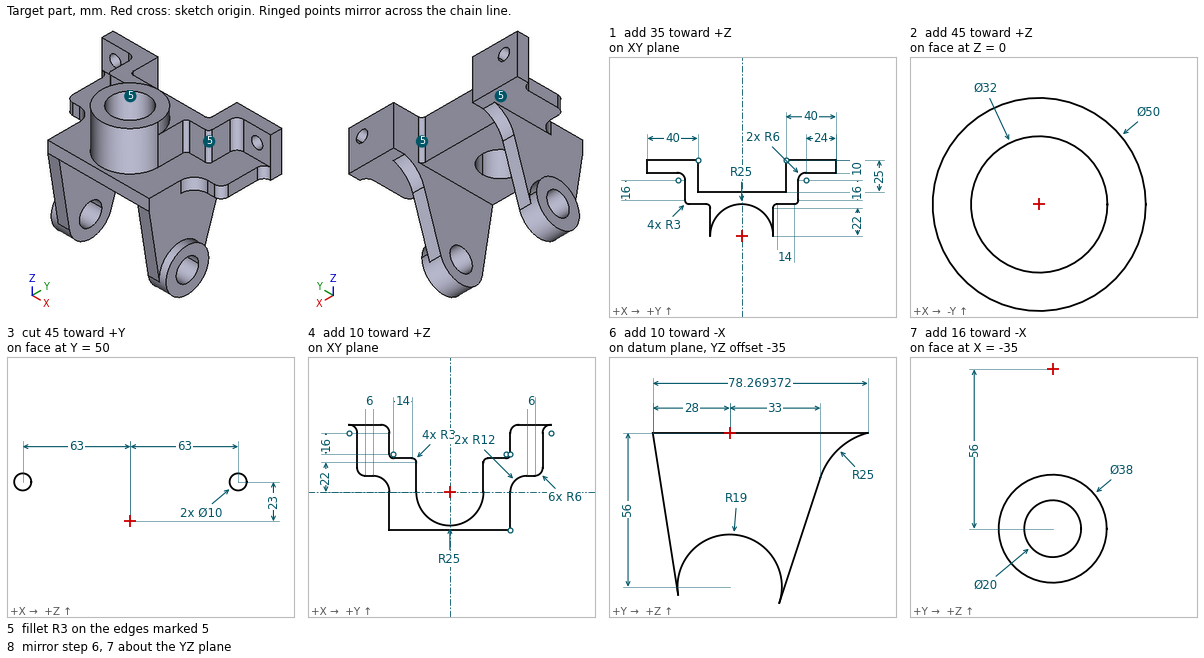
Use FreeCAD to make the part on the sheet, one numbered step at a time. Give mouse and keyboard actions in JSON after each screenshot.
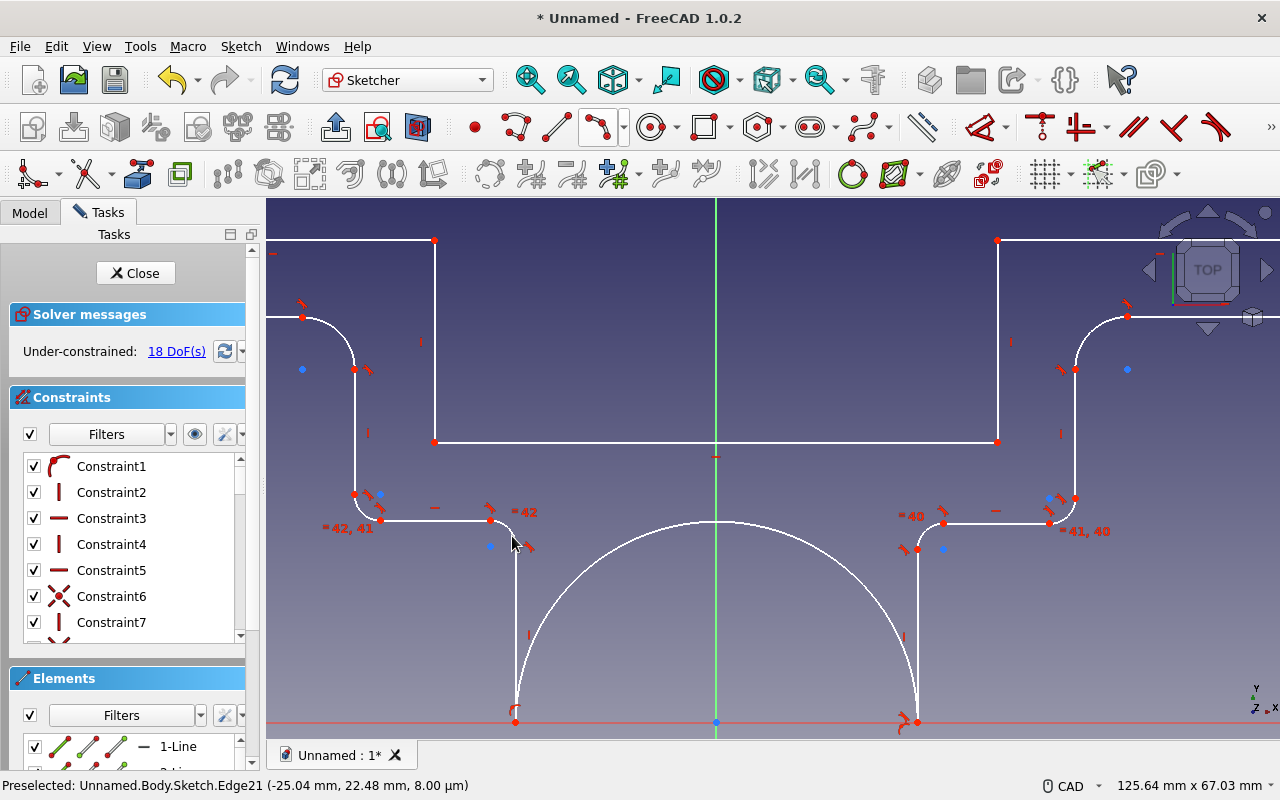
{"action": "left_click", "coordinate": [1104, 323]}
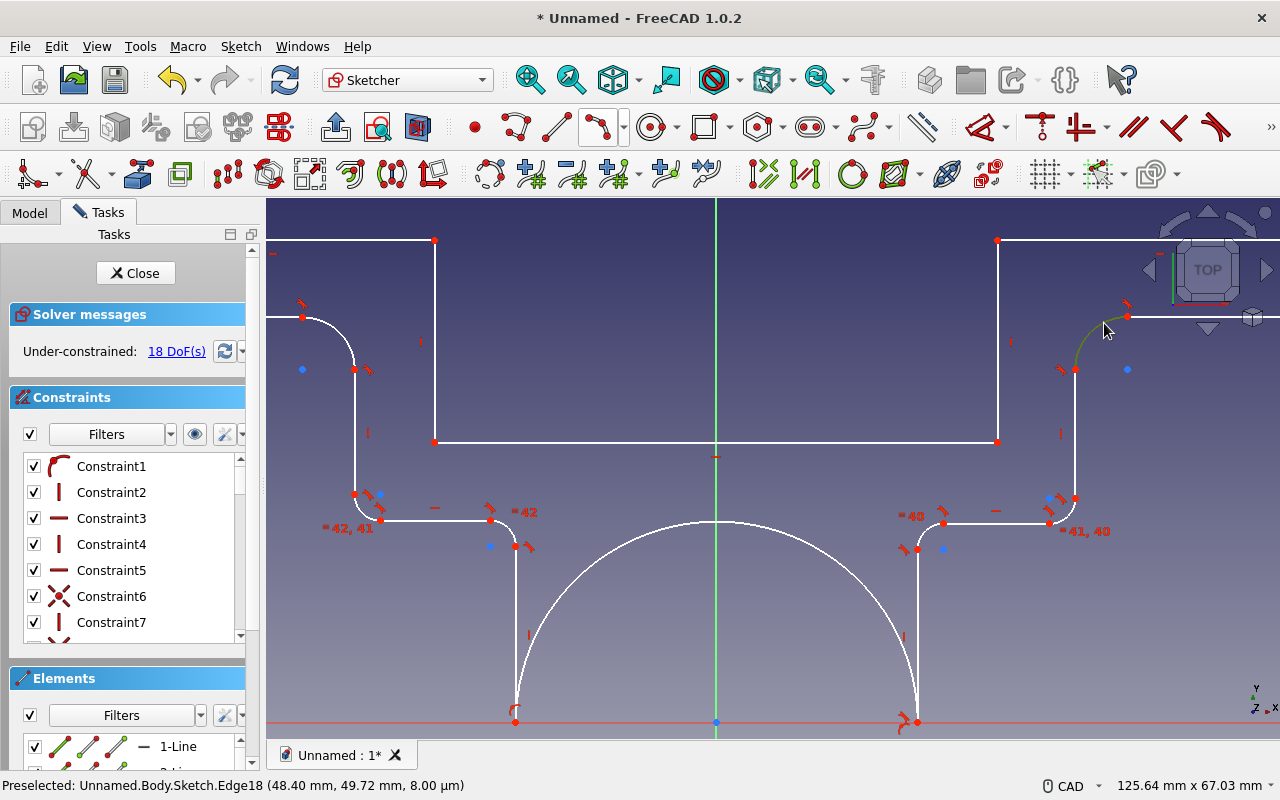
{"action": "left_click", "coordinate": [349, 346]}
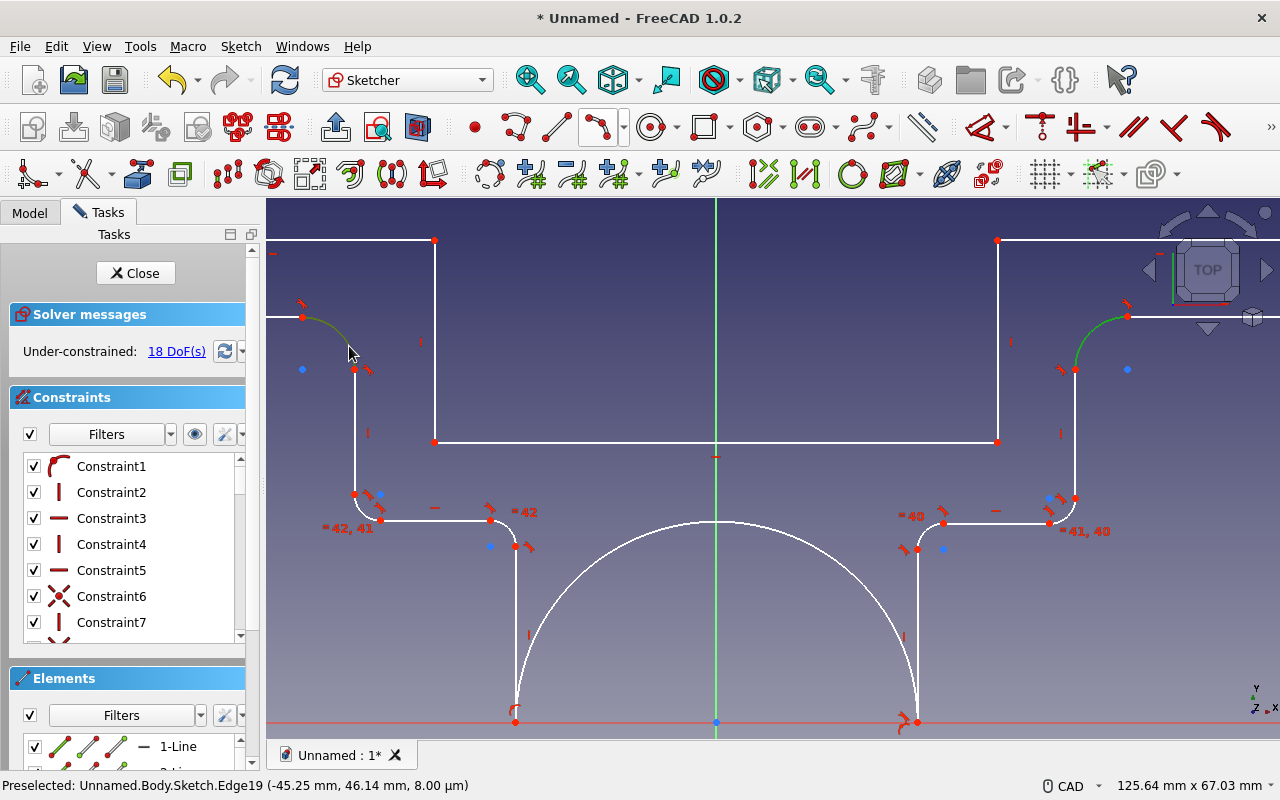
{"action": "key", "text": "e"}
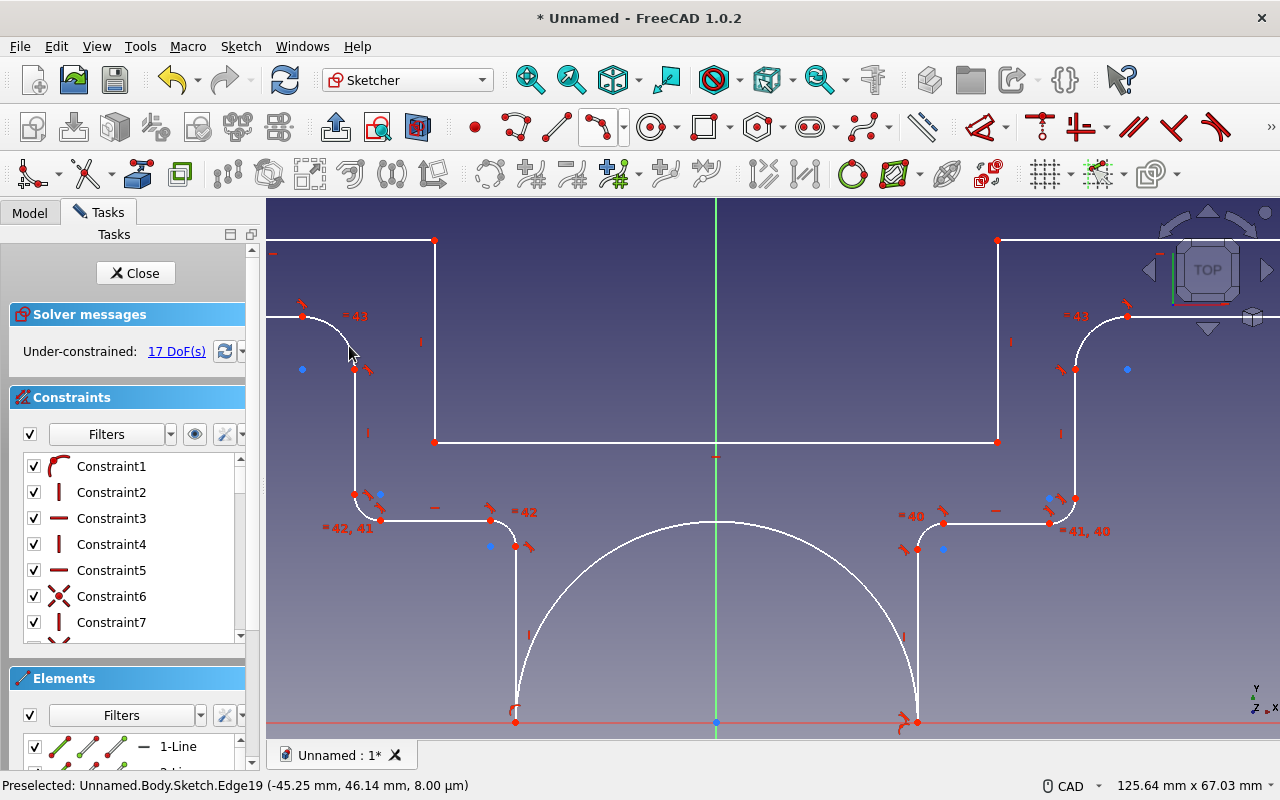
{"action": "scroll", "coordinate": [695, 459], "scroll_direction": "down", "scroll_amount": 4}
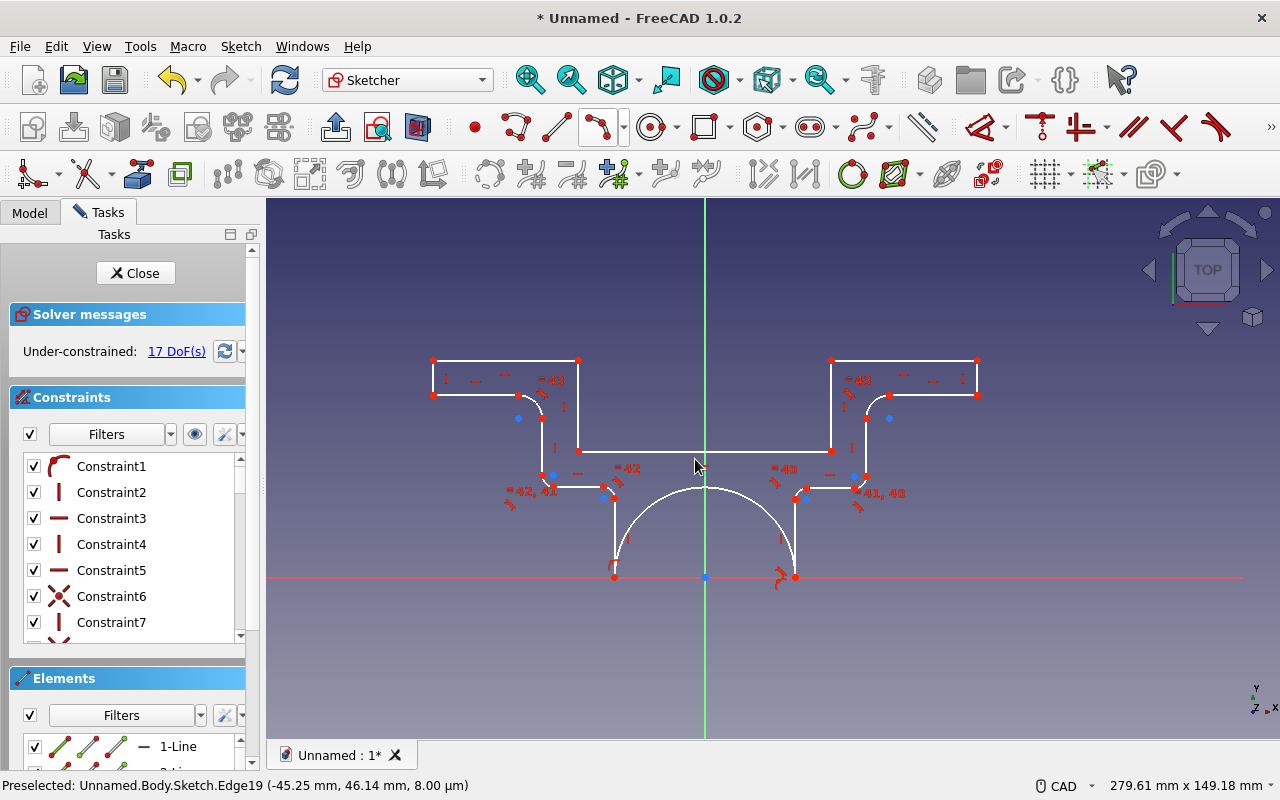
{"action": "left_click", "coordinate": [705, 578]}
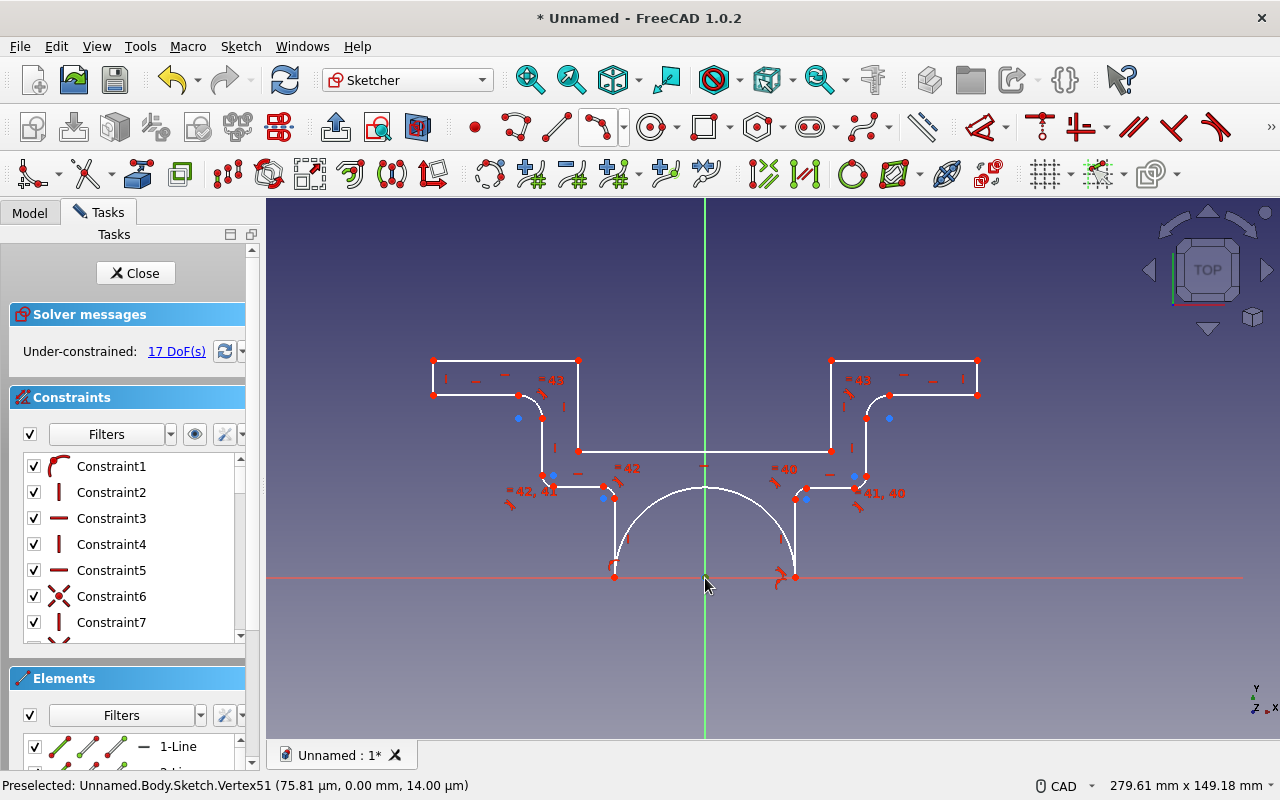
{"action": "left_click", "coordinate": [705, 676]}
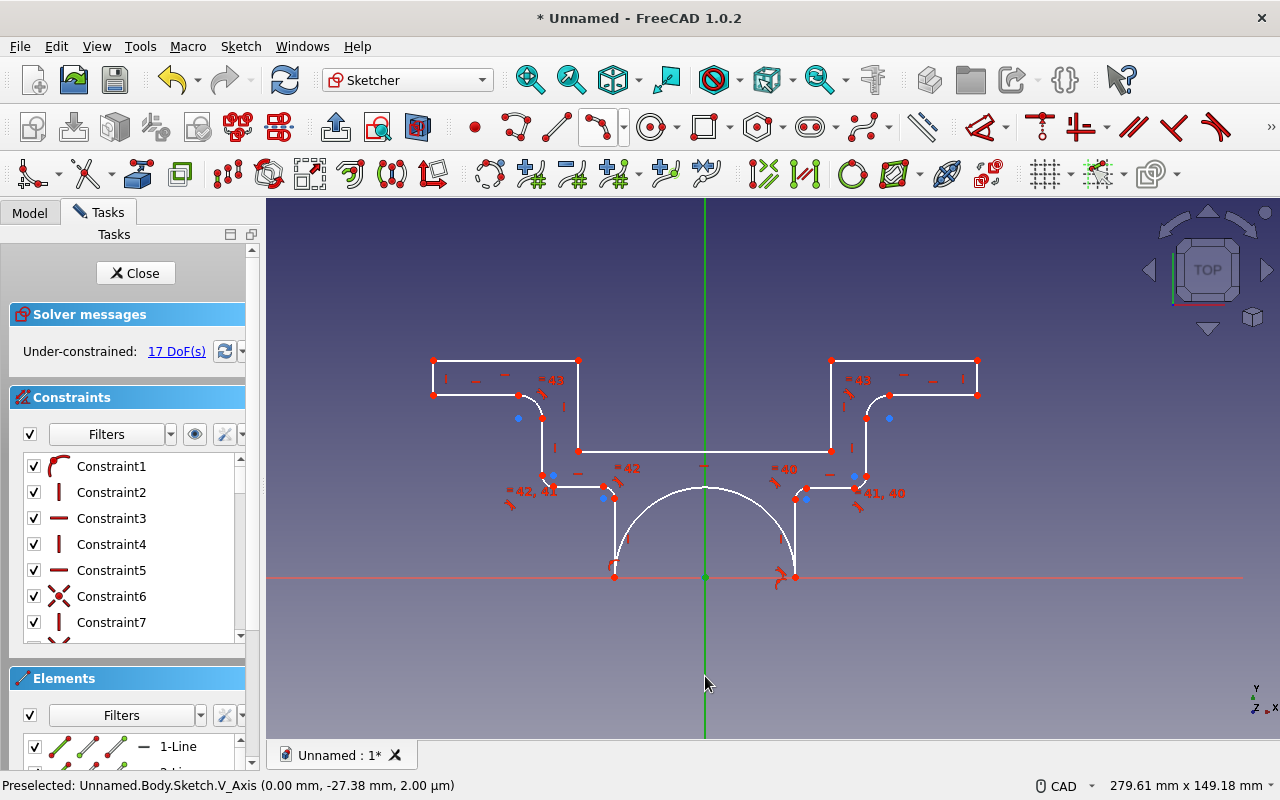
{"action": "left_click", "coordinate": [1040, 128]}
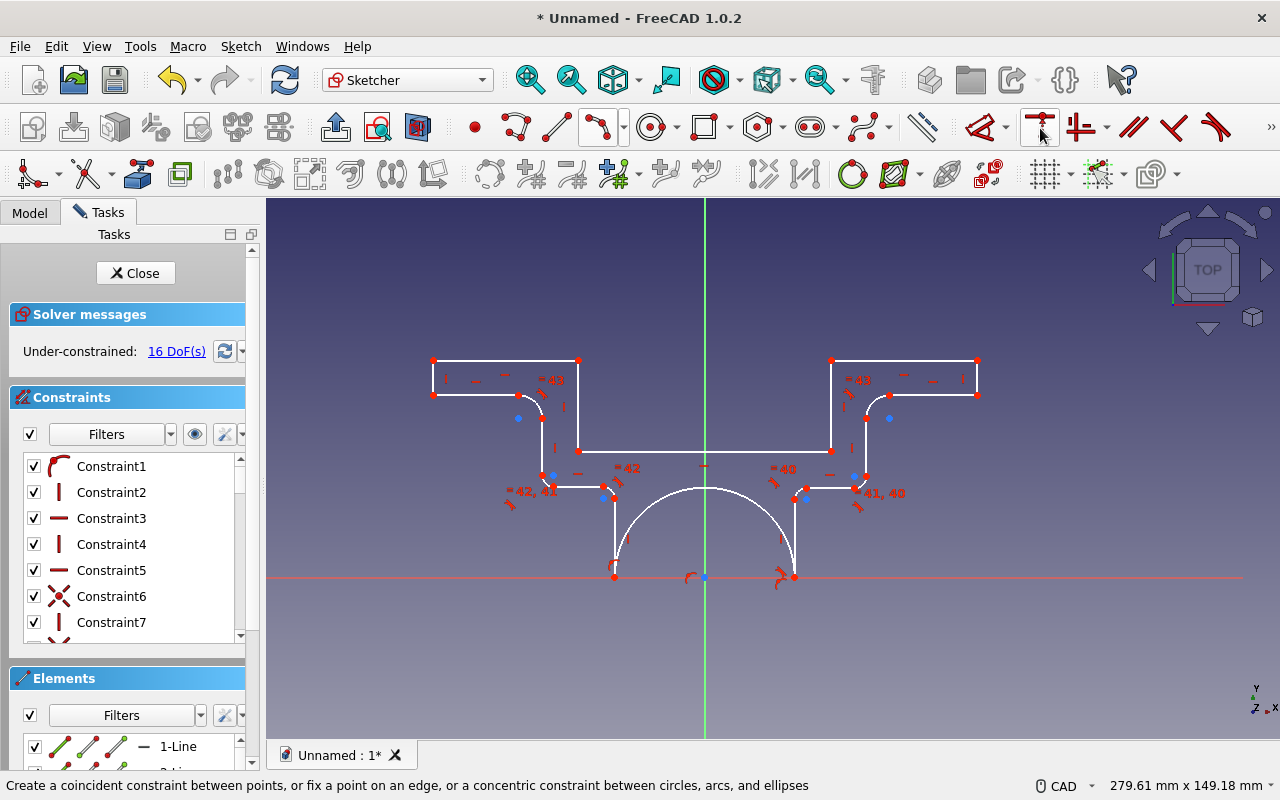
{"action": "left_click", "coordinate": [890, 419]}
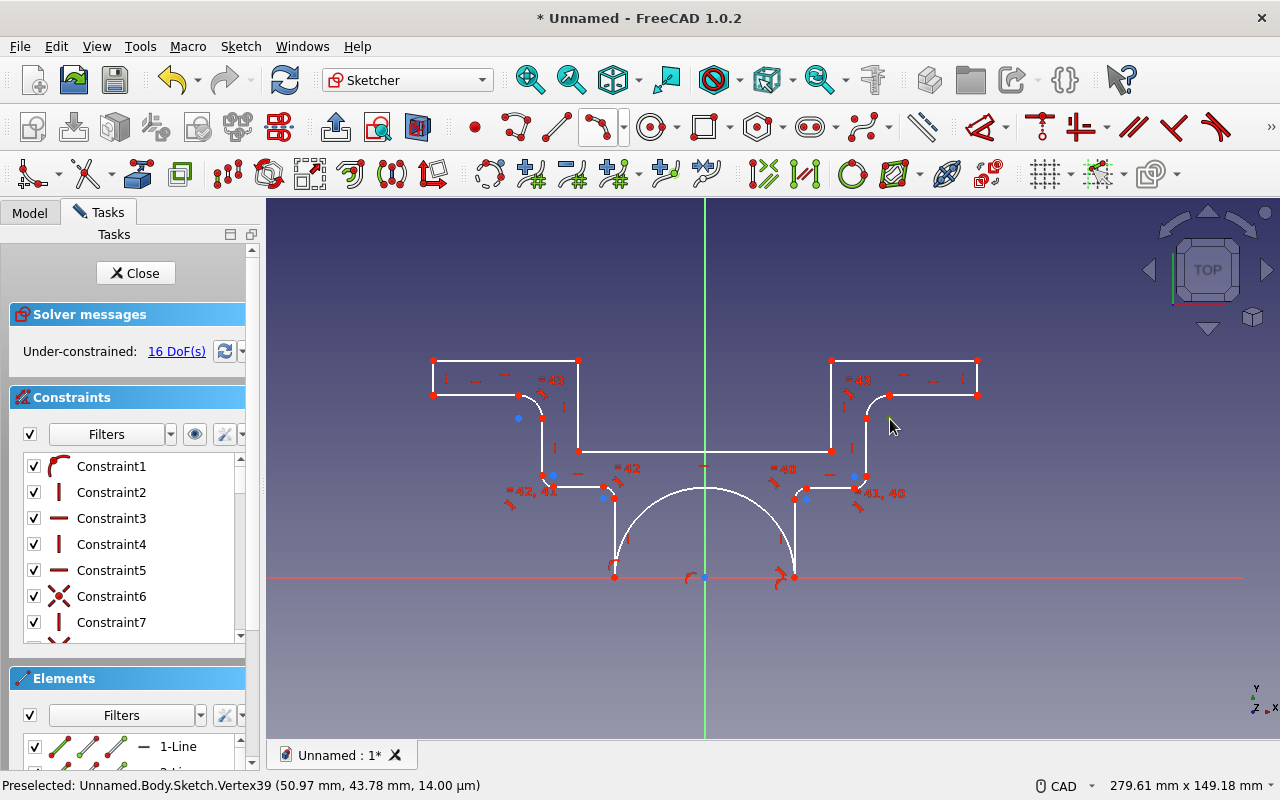
{"action": "left_click", "coordinate": [519, 419]}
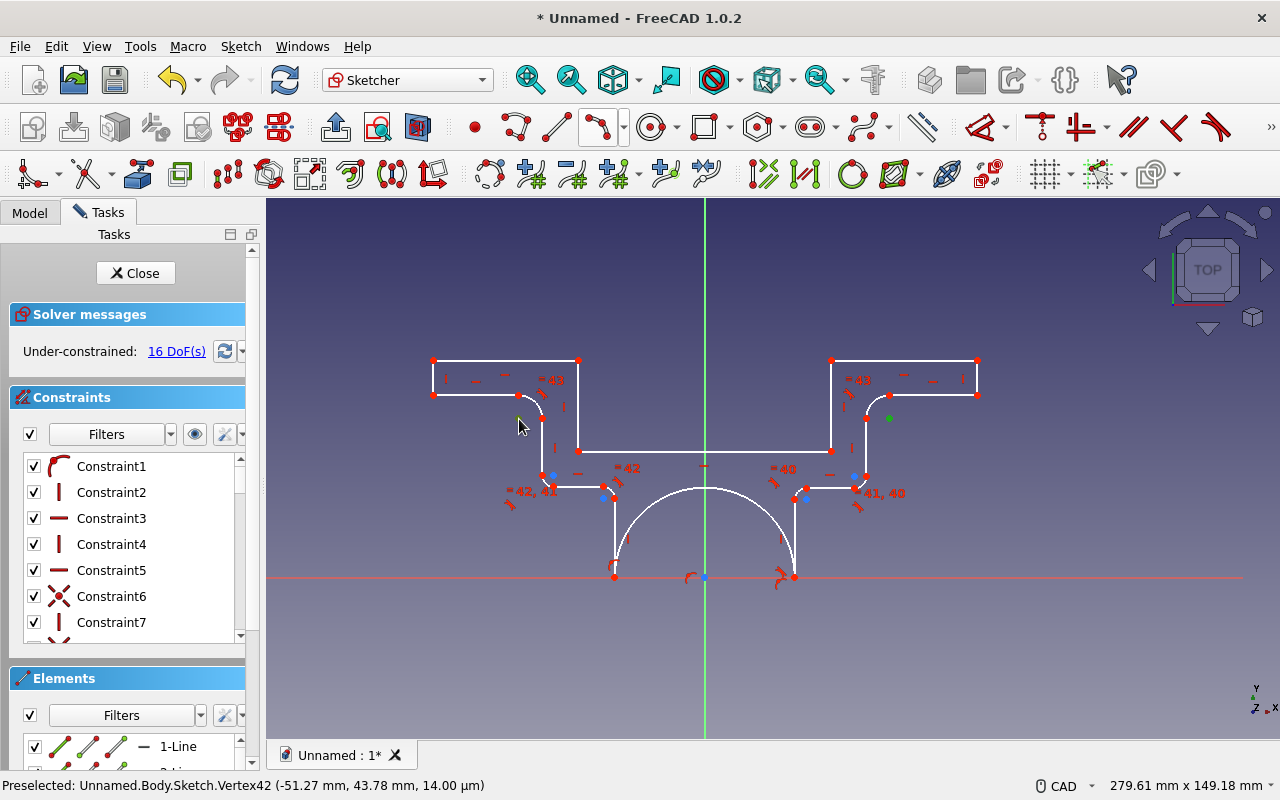
{"action": "left_click", "coordinate": [705, 676]}